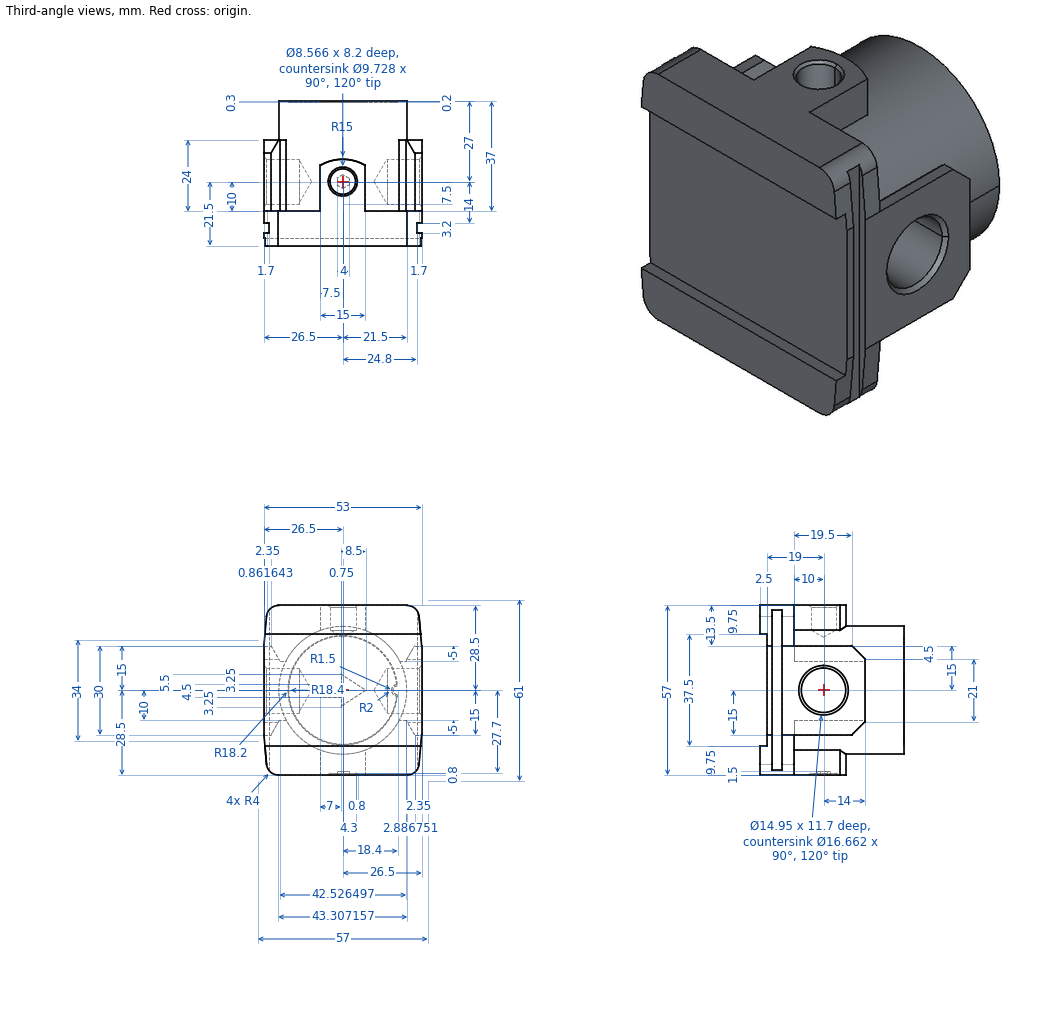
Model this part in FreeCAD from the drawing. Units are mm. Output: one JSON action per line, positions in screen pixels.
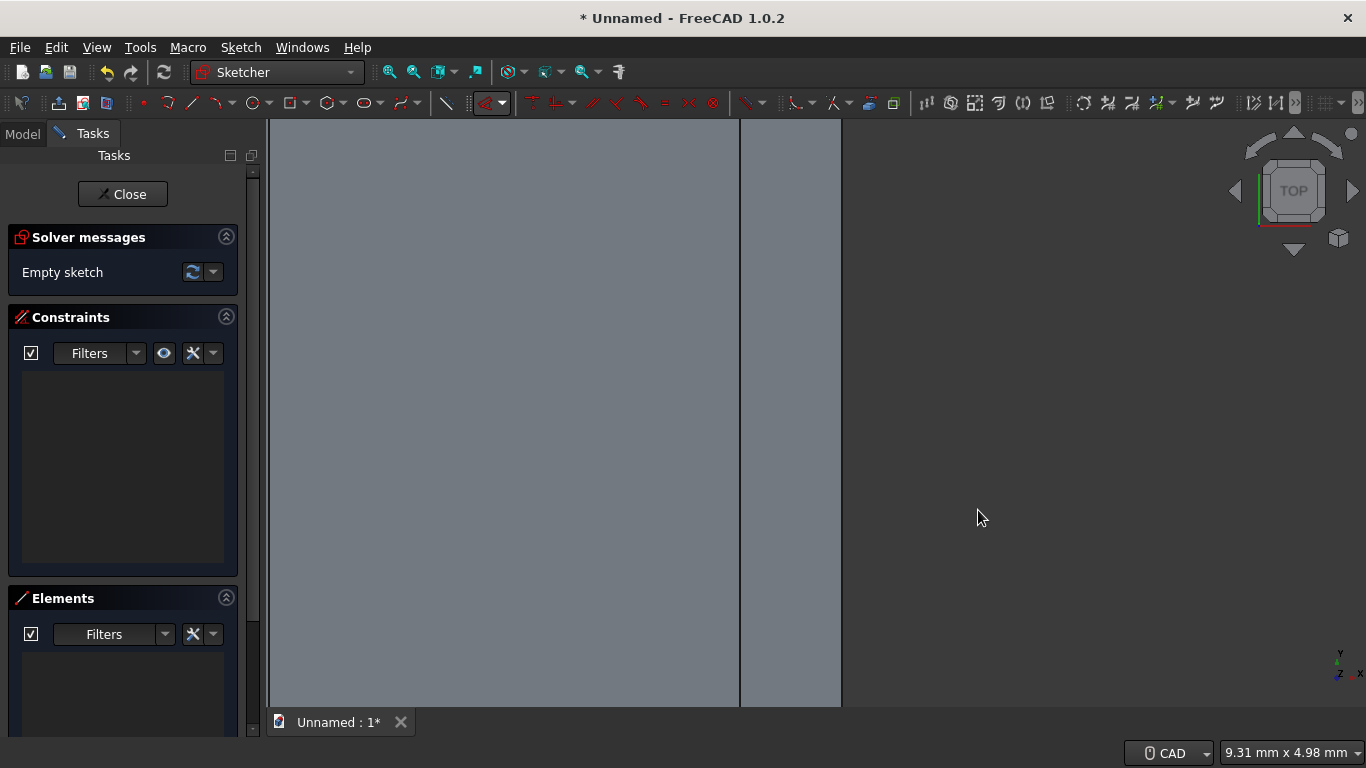
{"action": "key", "text": "g r"}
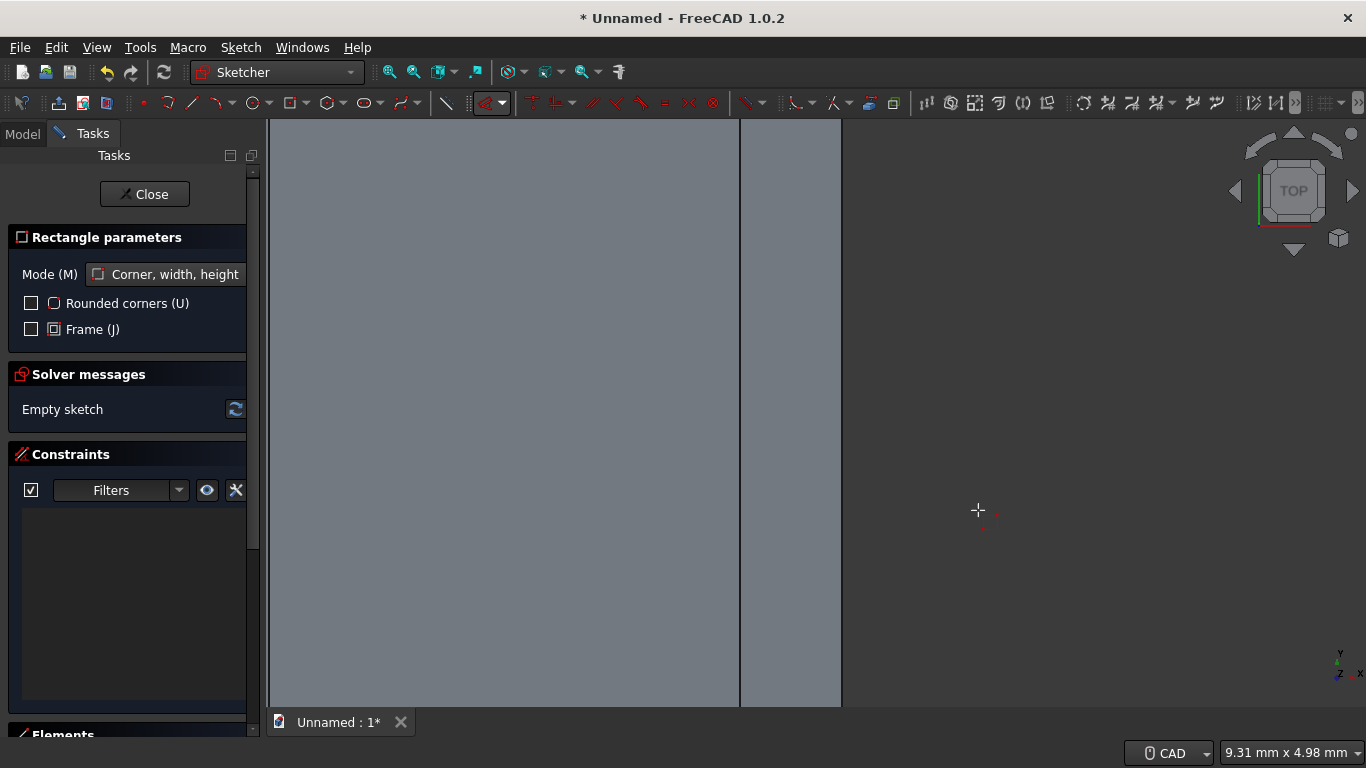
{"action": "left_click", "coordinate": [641, 202]}
{"action": "mouse_move", "coordinate": [842, 580]}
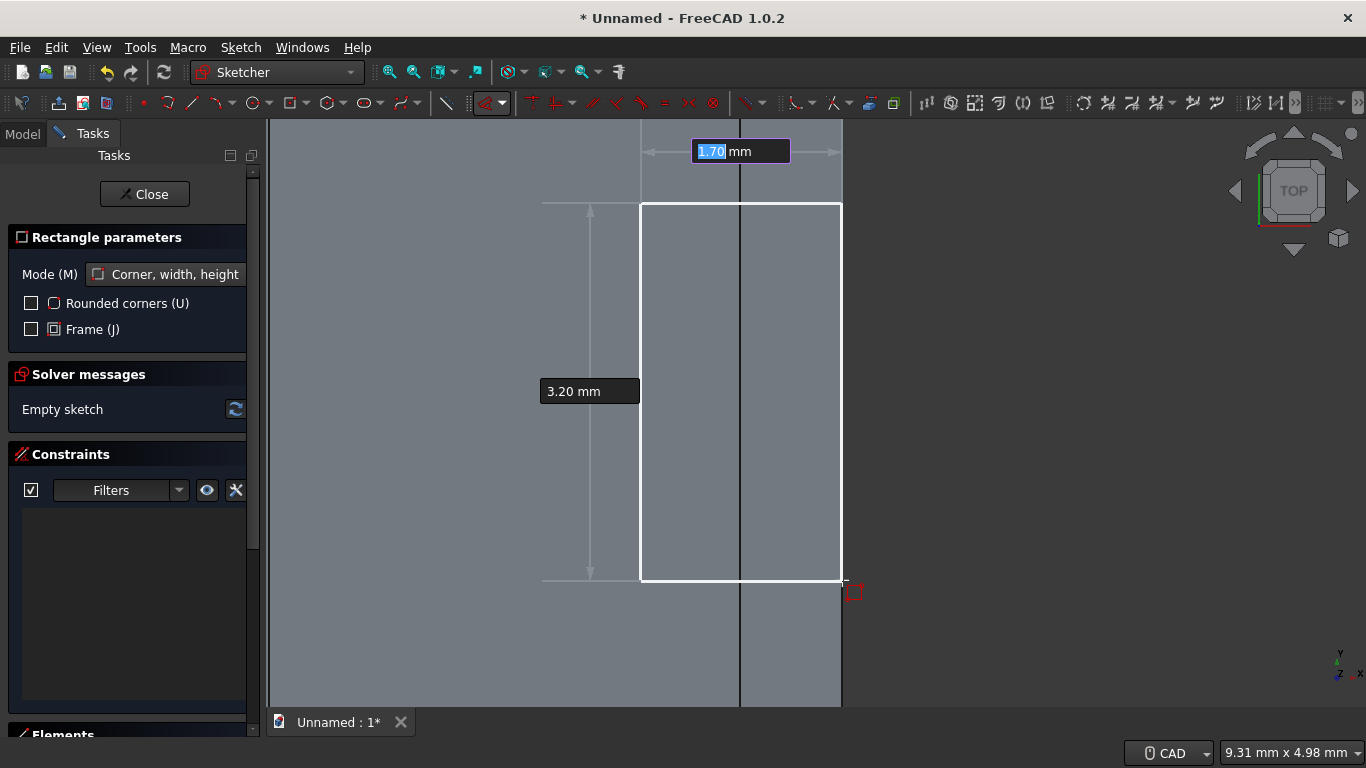
{"action": "type", "text": "1.7"}
{"action": "key", "text": "Tab"}
{"action": "type", "text": "3.2"}
{"action": "key", "text": "Return"}
{"action": "key", "text": "Escape"}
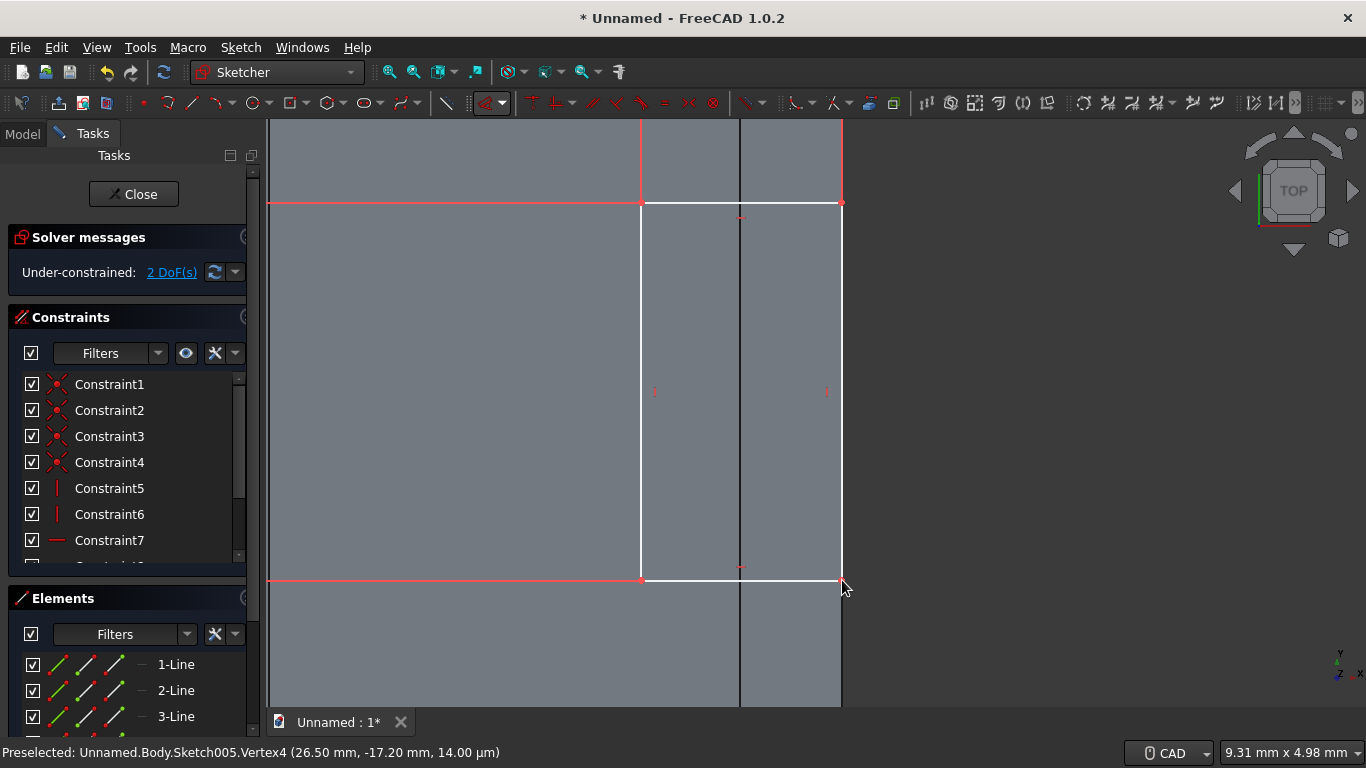
{"action": "left_click", "coordinate": [641, 203]}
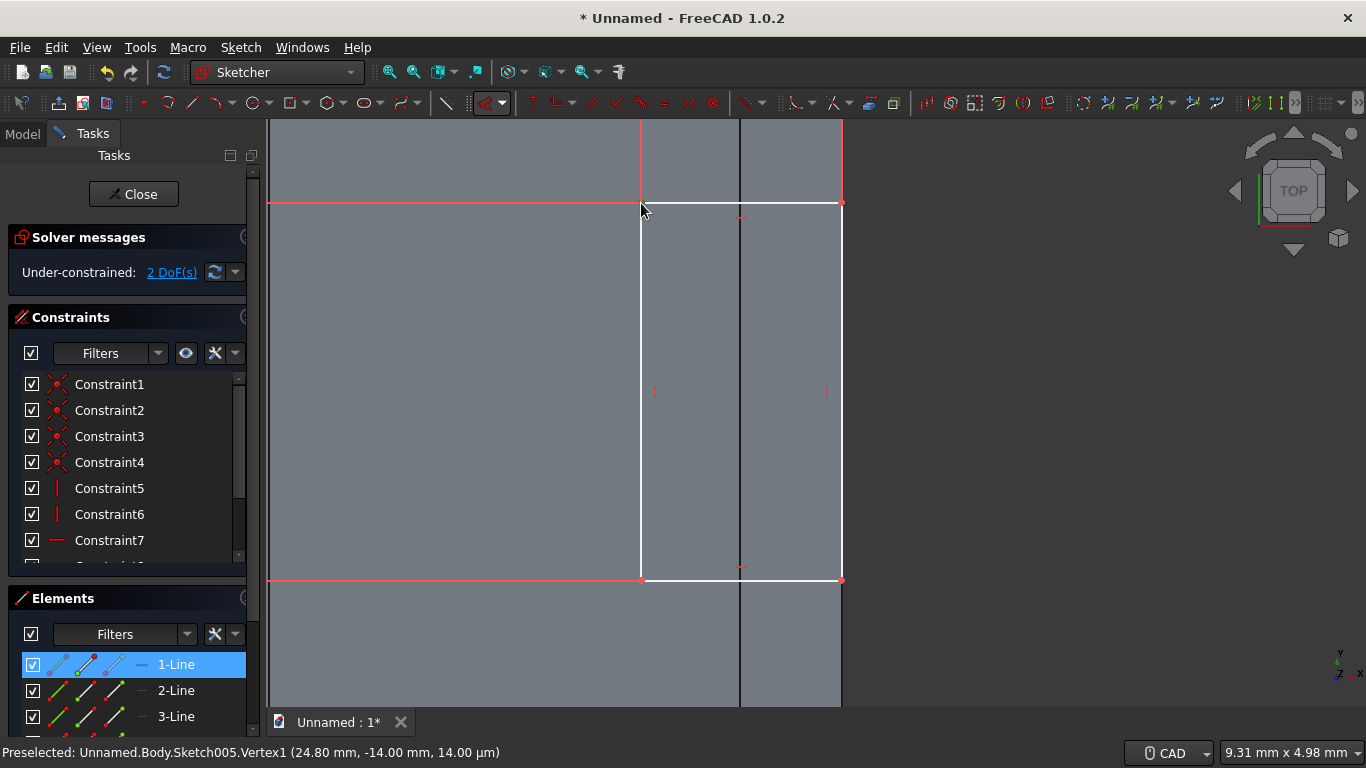
{"action": "key", "text": "i"}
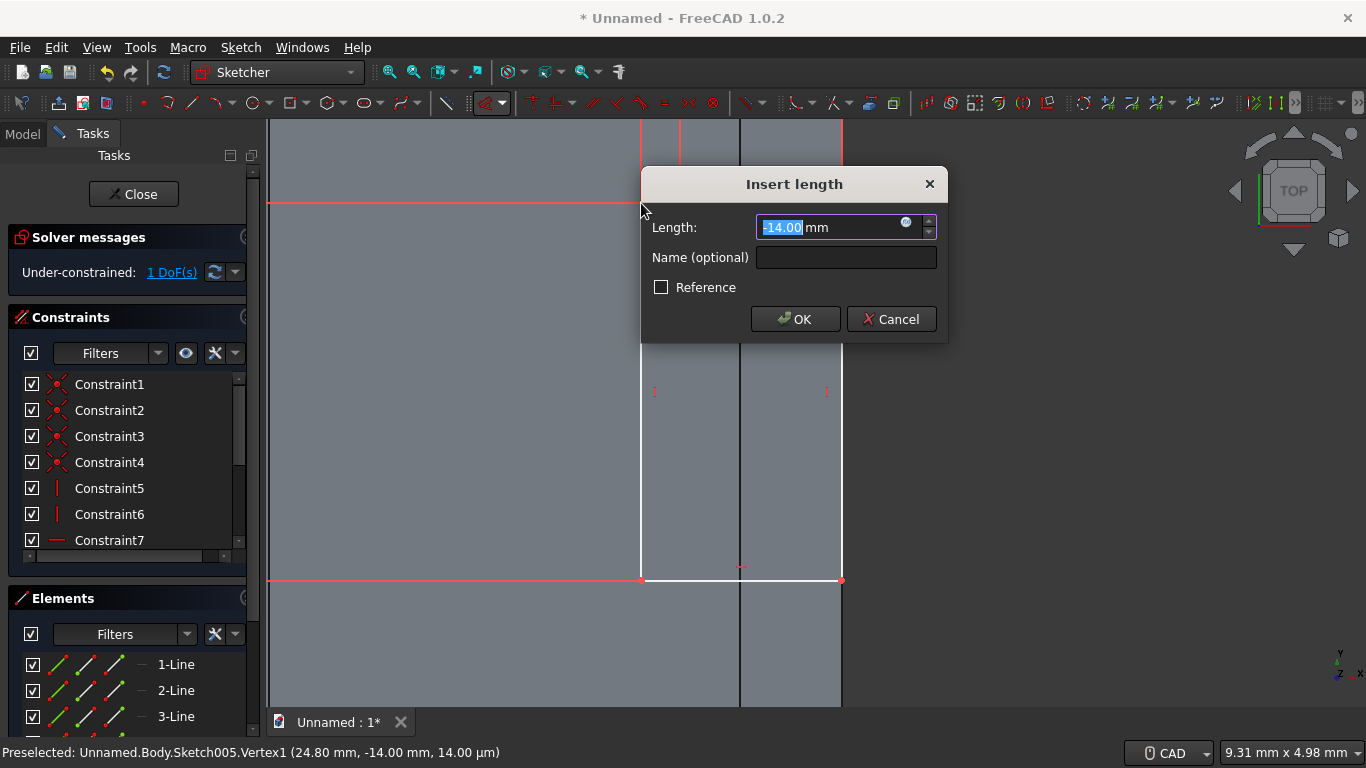
{"action": "type", "text": "-14"}
{"action": "key", "text": "Return"}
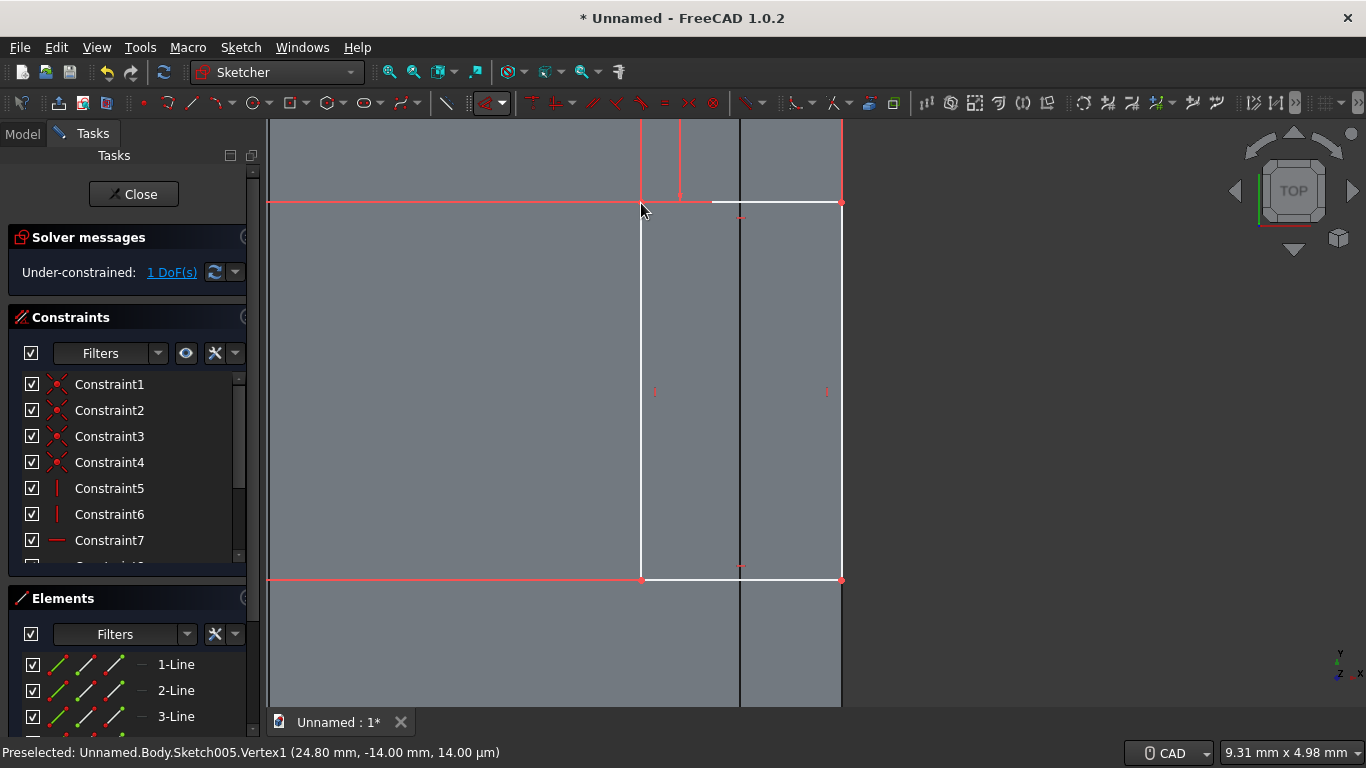
{"action": "left_click", "coordinate": [641, 202]}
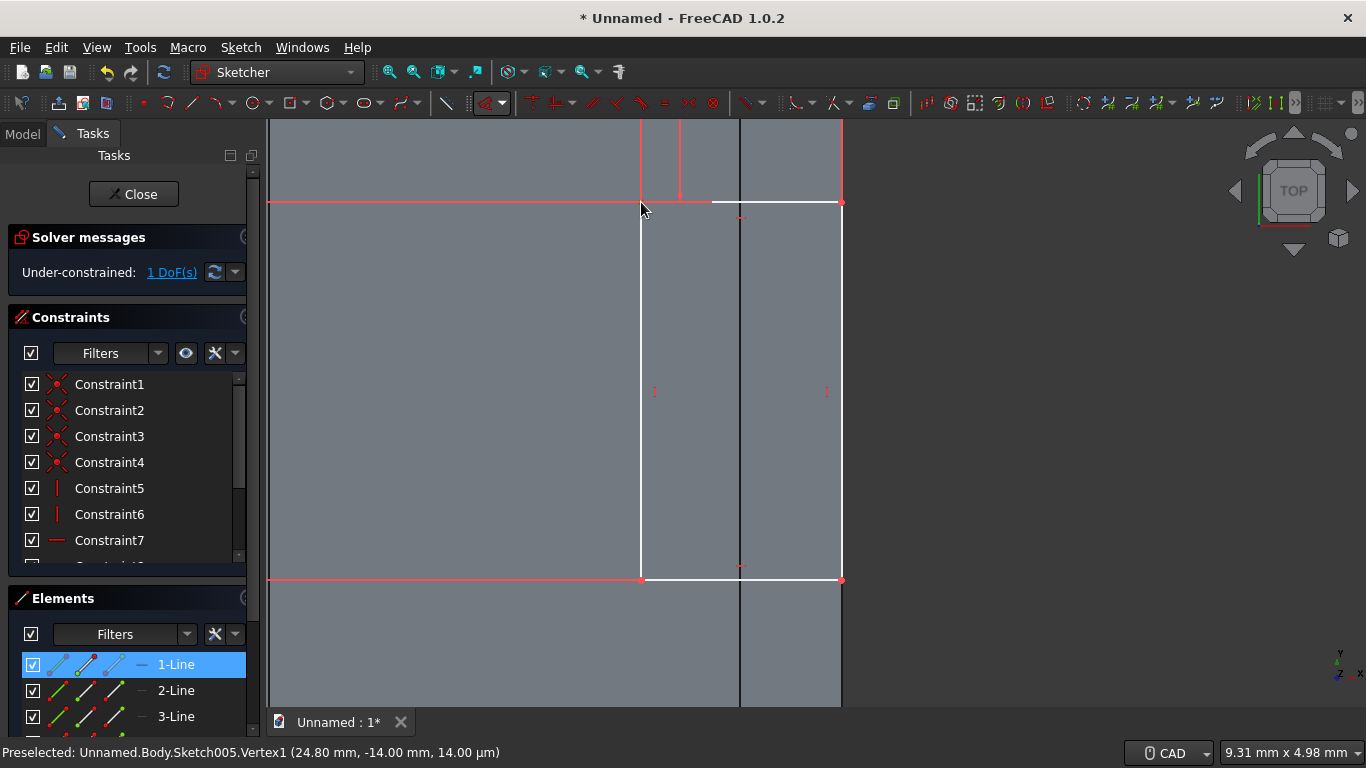
{"action": "key", "text": "l"}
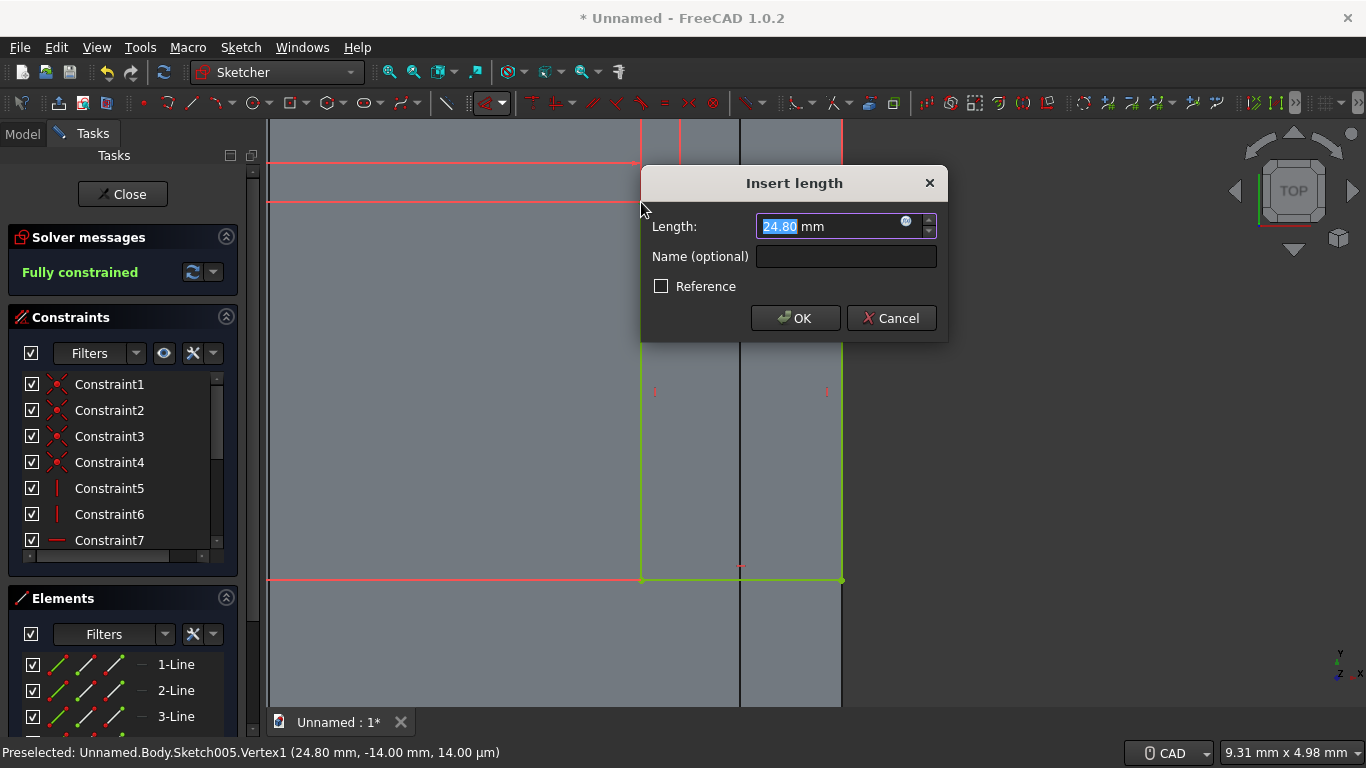
{"action": "type", "text": "24.8"}
{"action": "key", "text": "Return"}